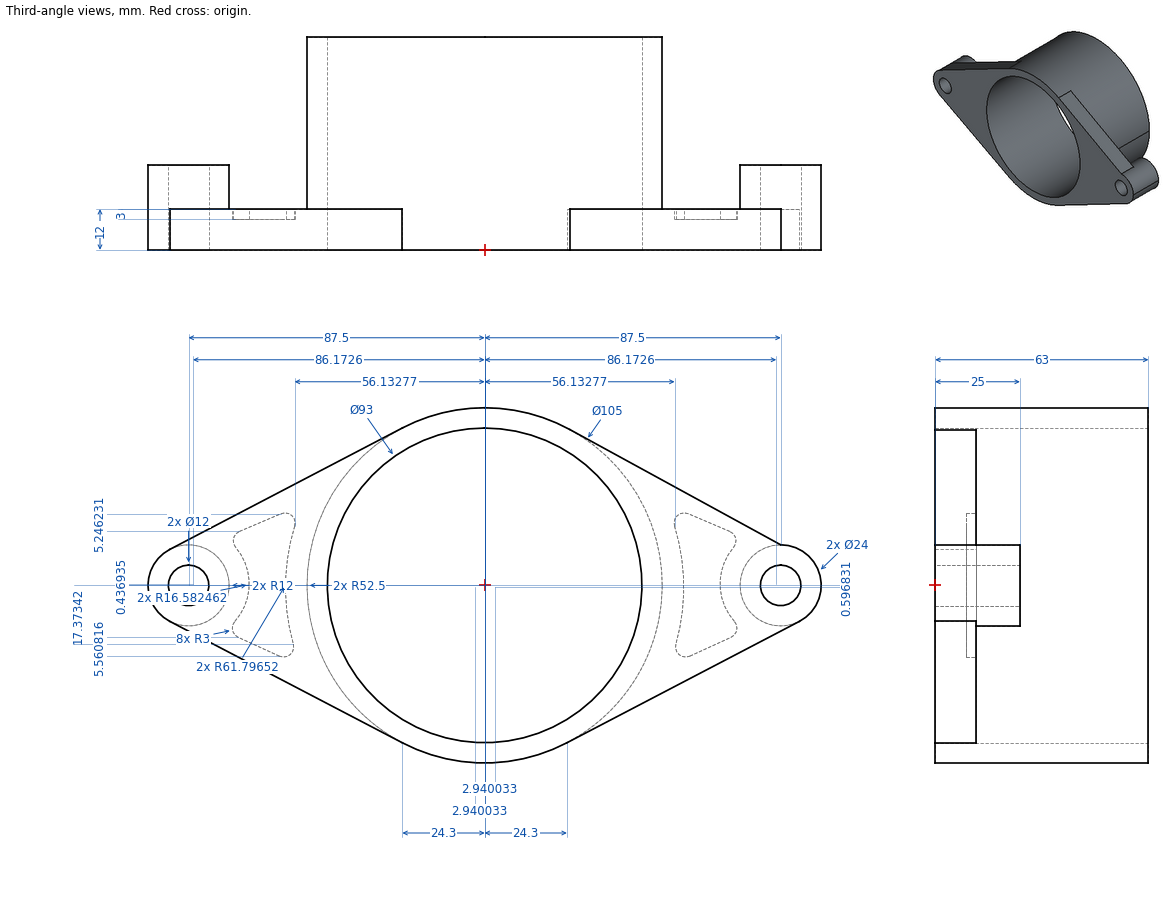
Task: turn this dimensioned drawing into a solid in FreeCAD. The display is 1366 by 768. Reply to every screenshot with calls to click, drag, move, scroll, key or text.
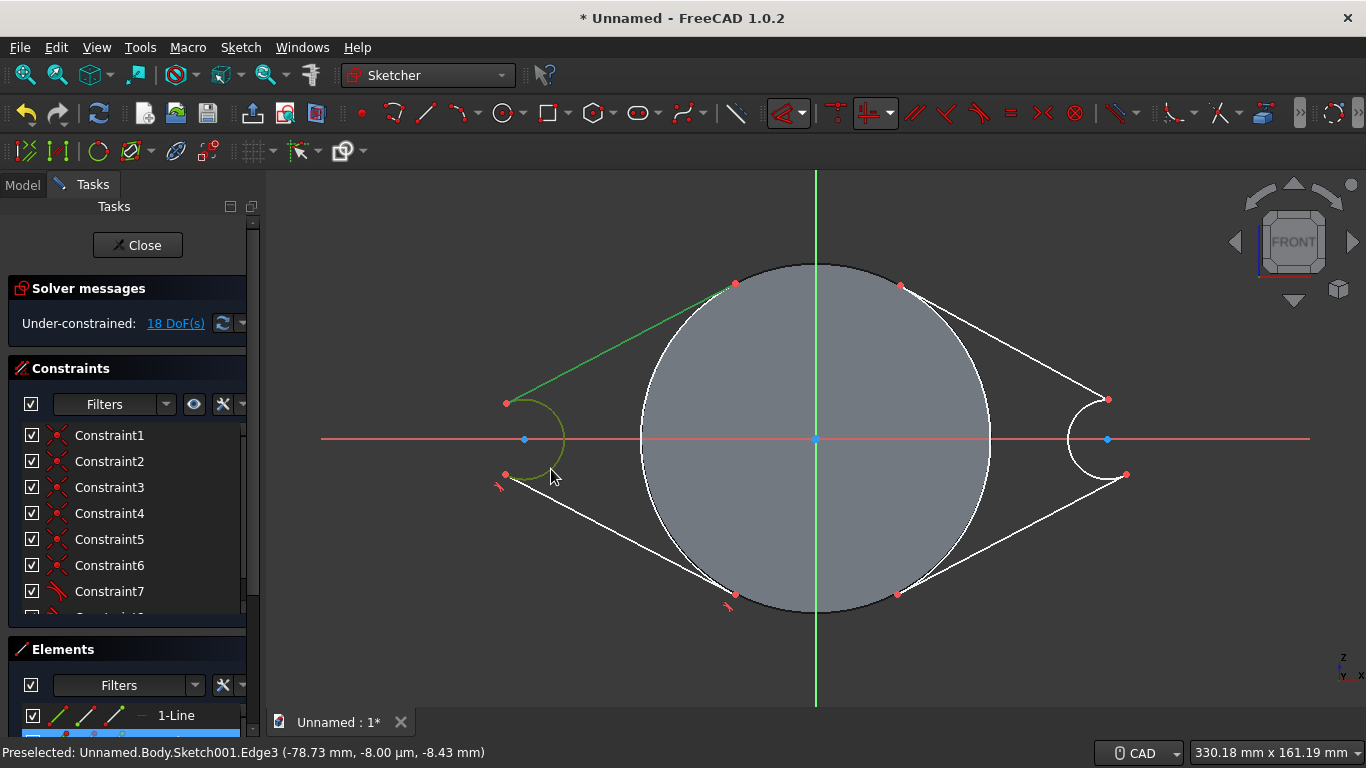
key(t)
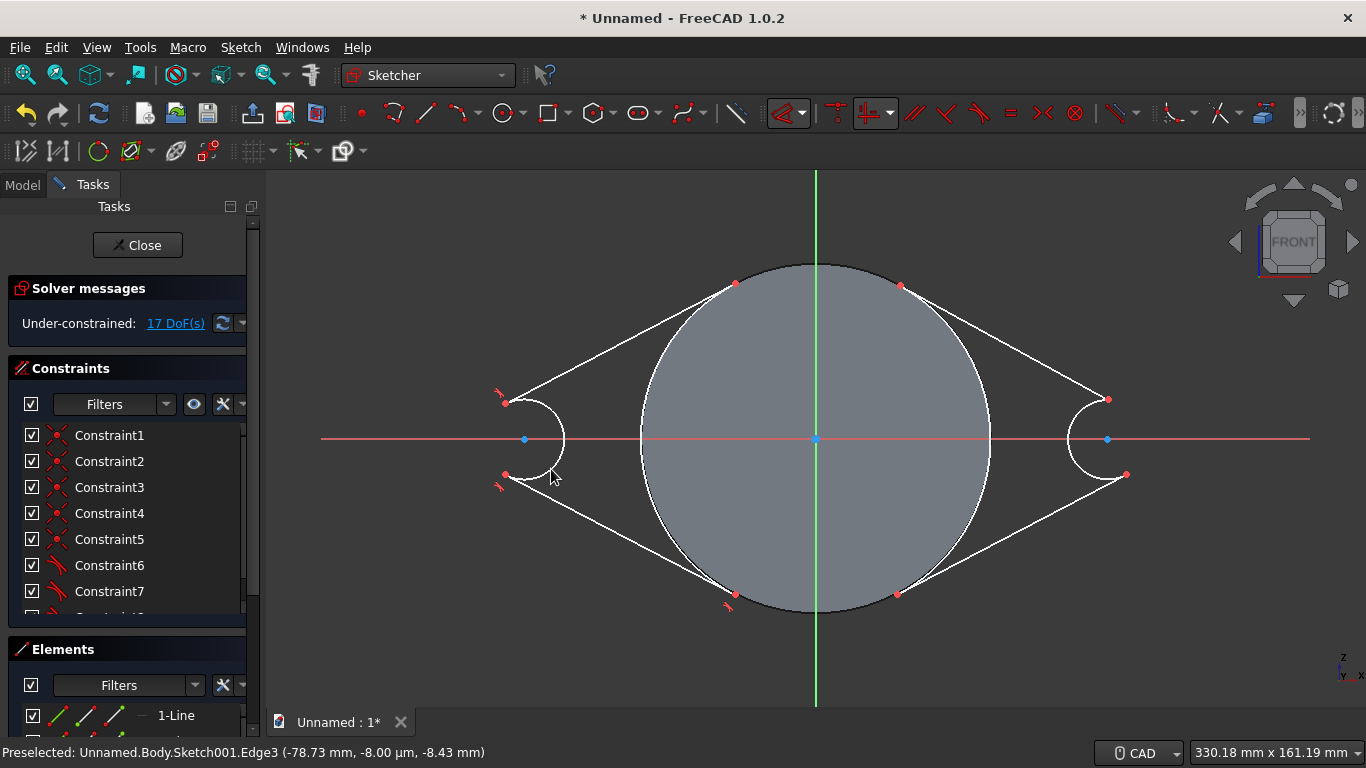
click(1057, 511)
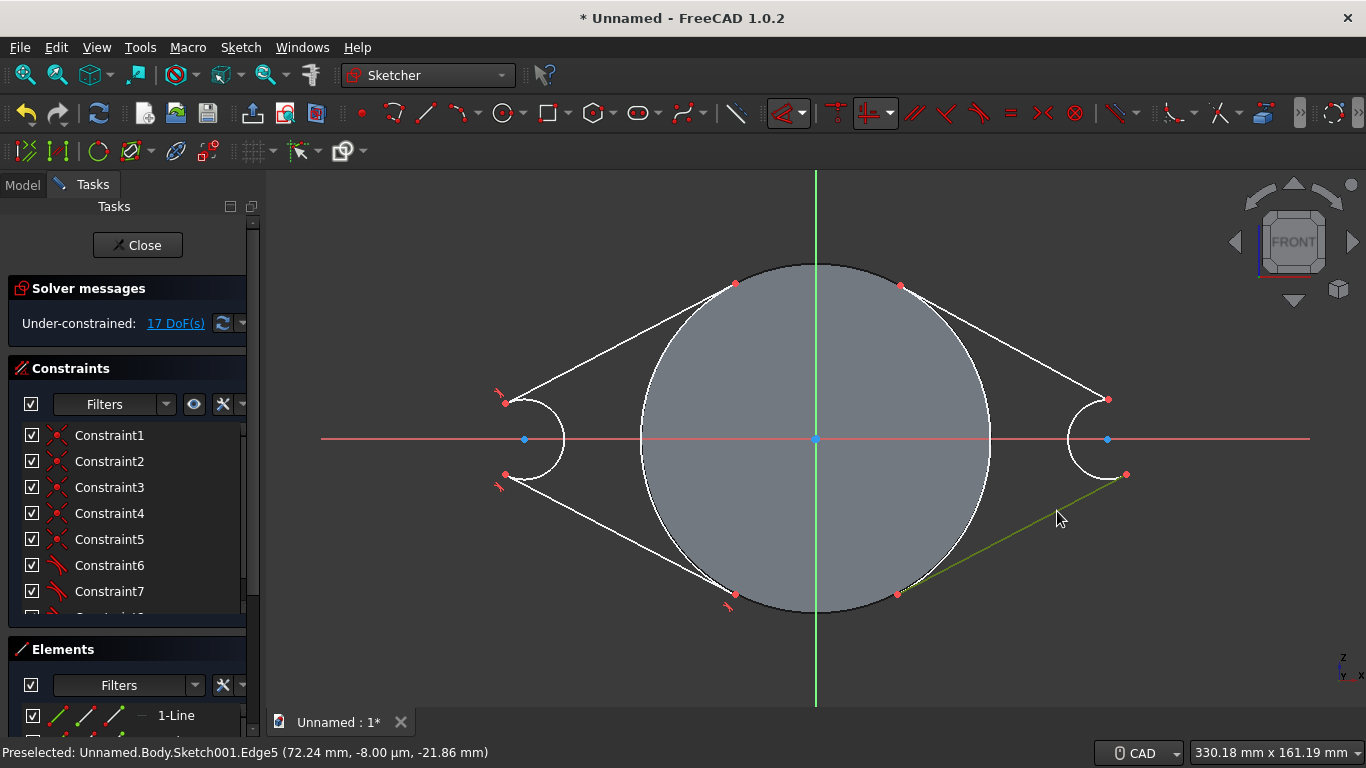
click(974, 514)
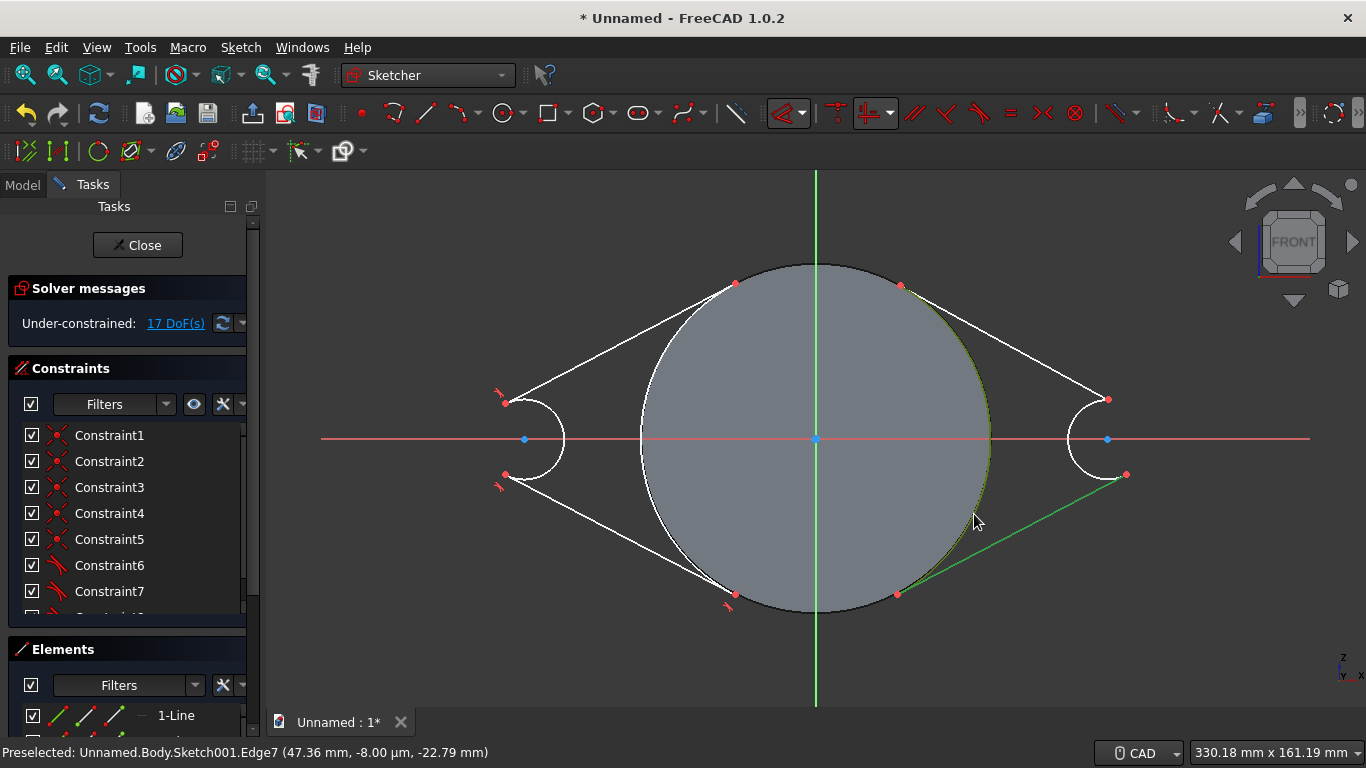
key(t)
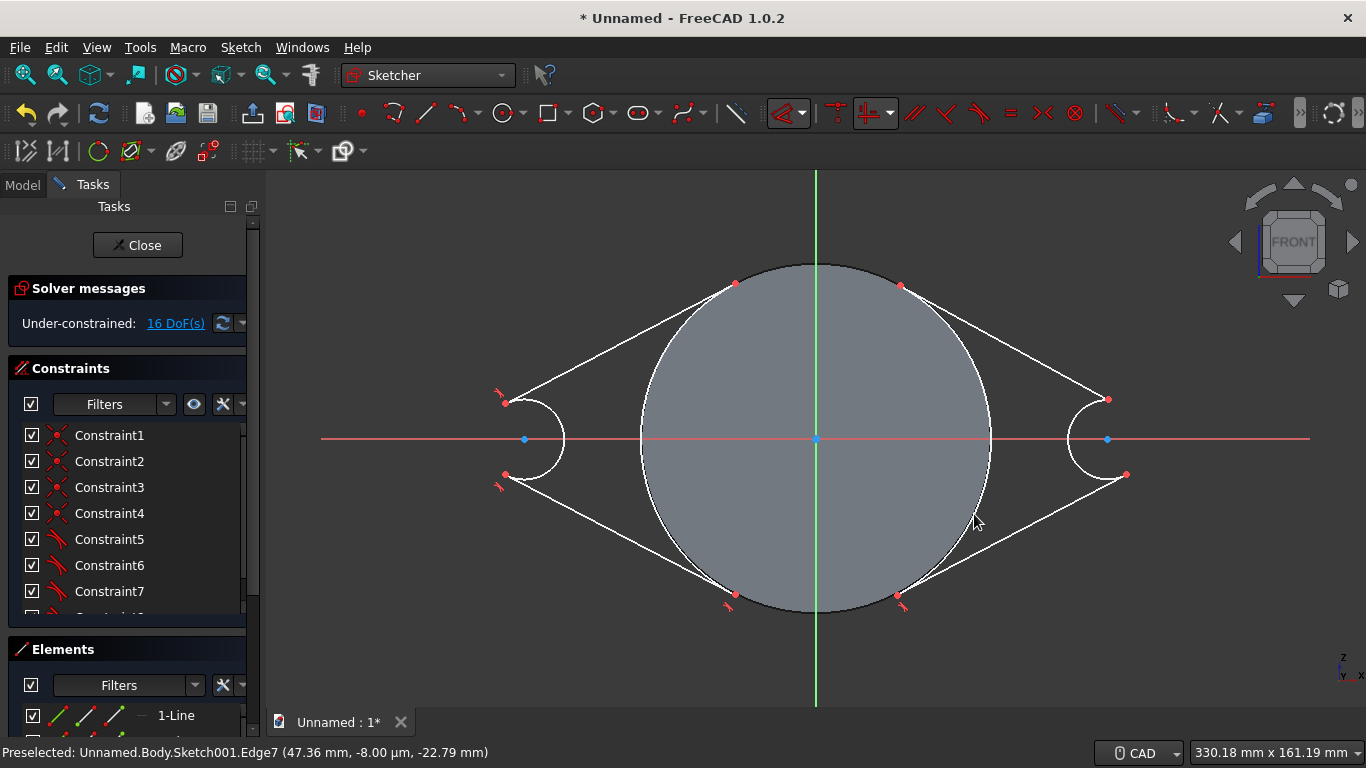
click(1057, 511)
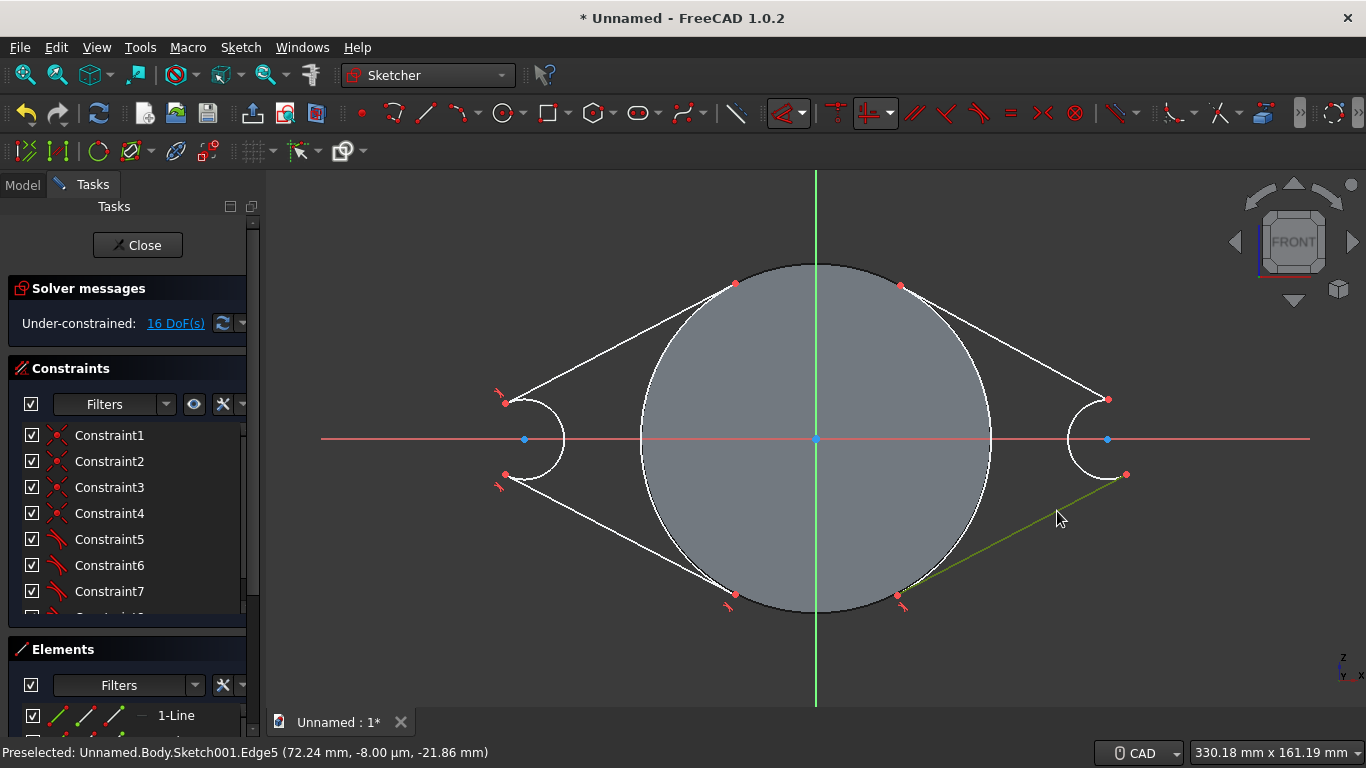
click(1073, 421)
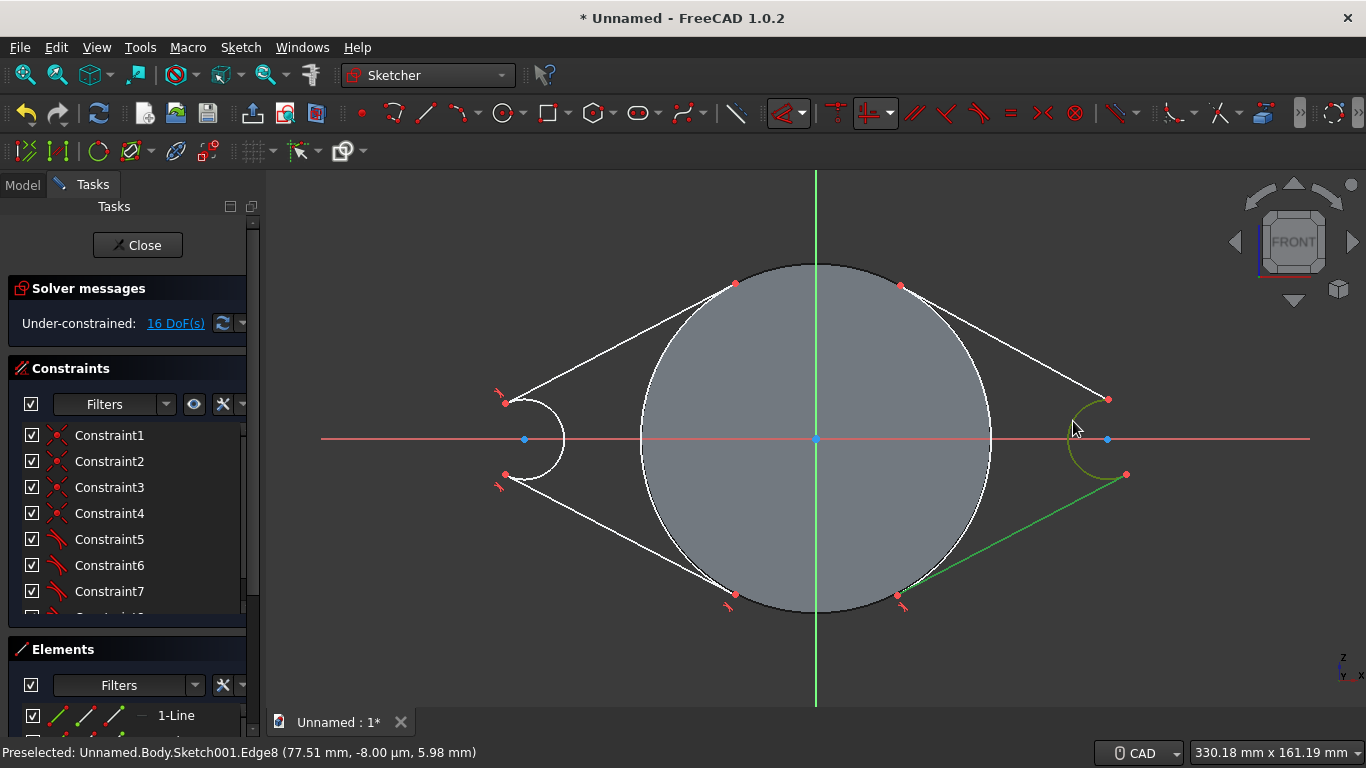
key(t)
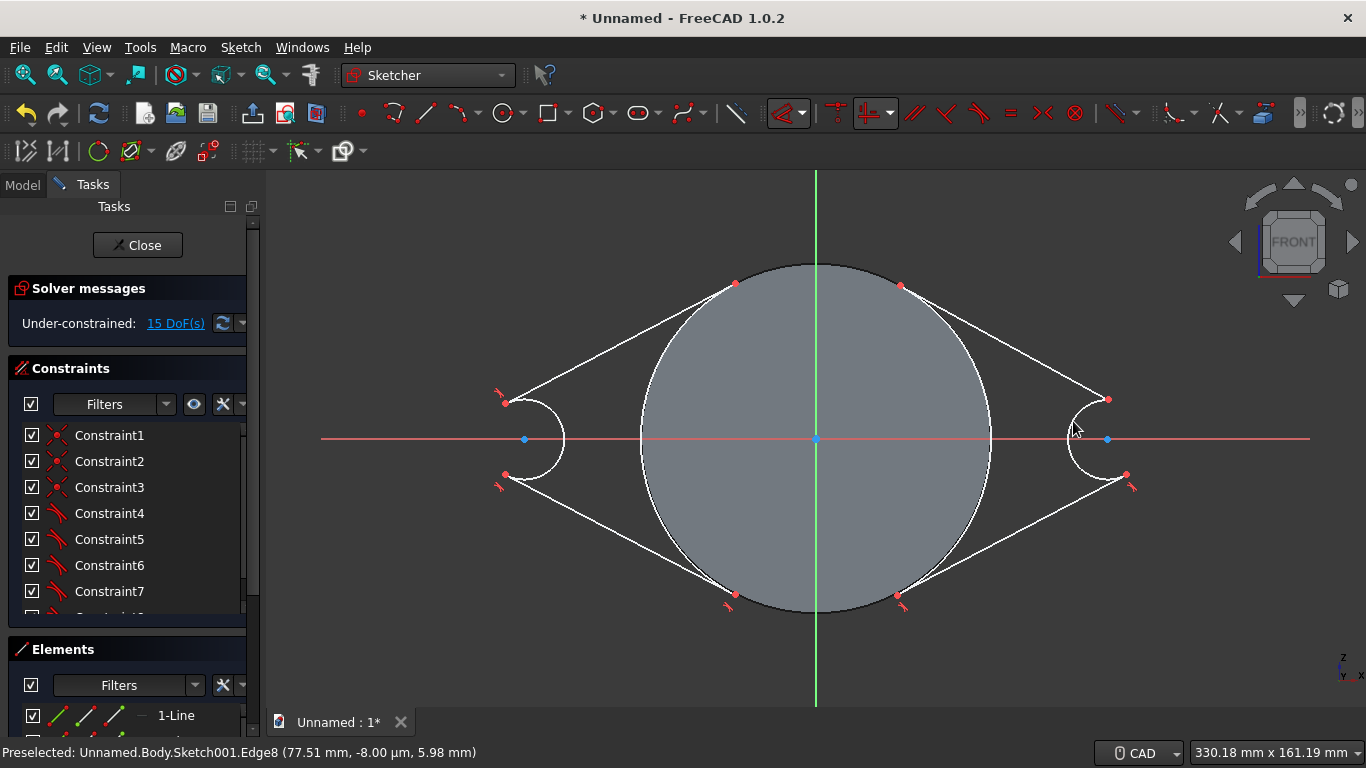
click(962, 320)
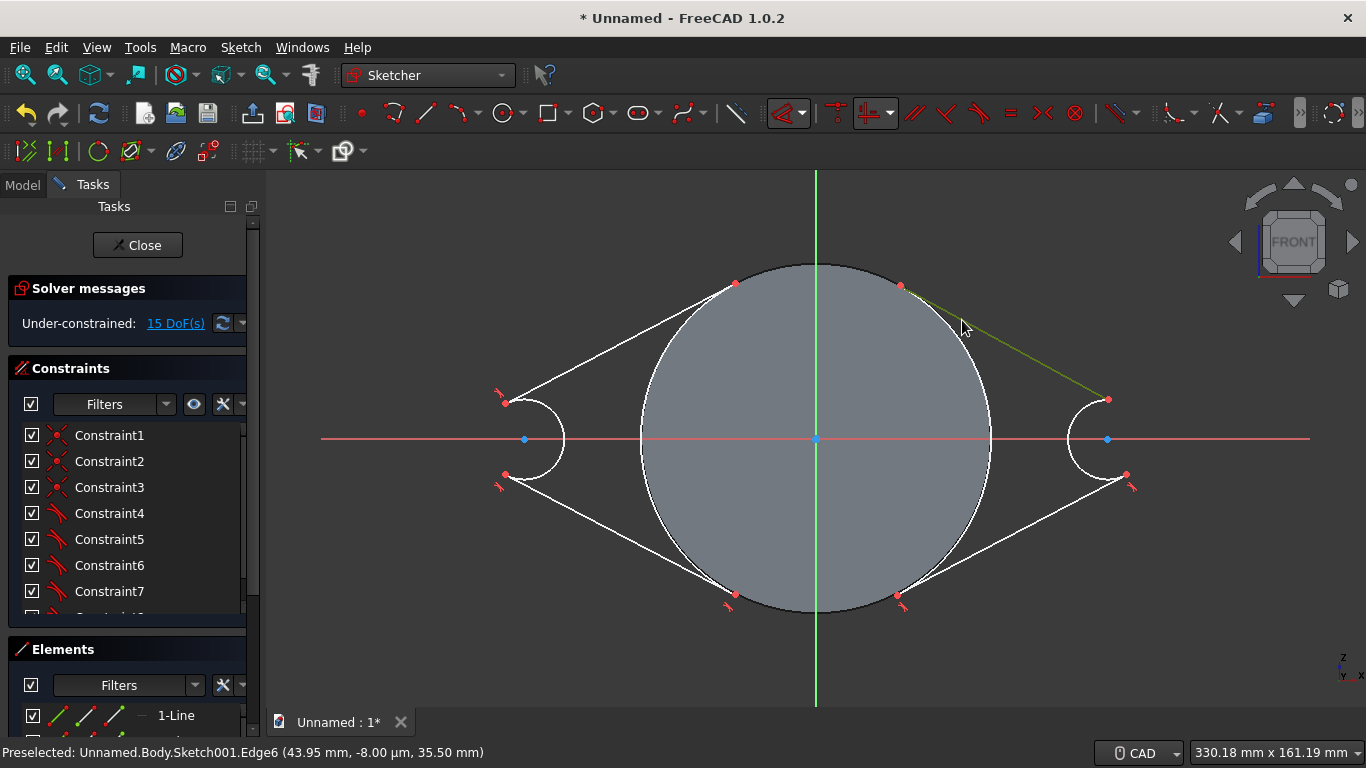
click(974, 515)